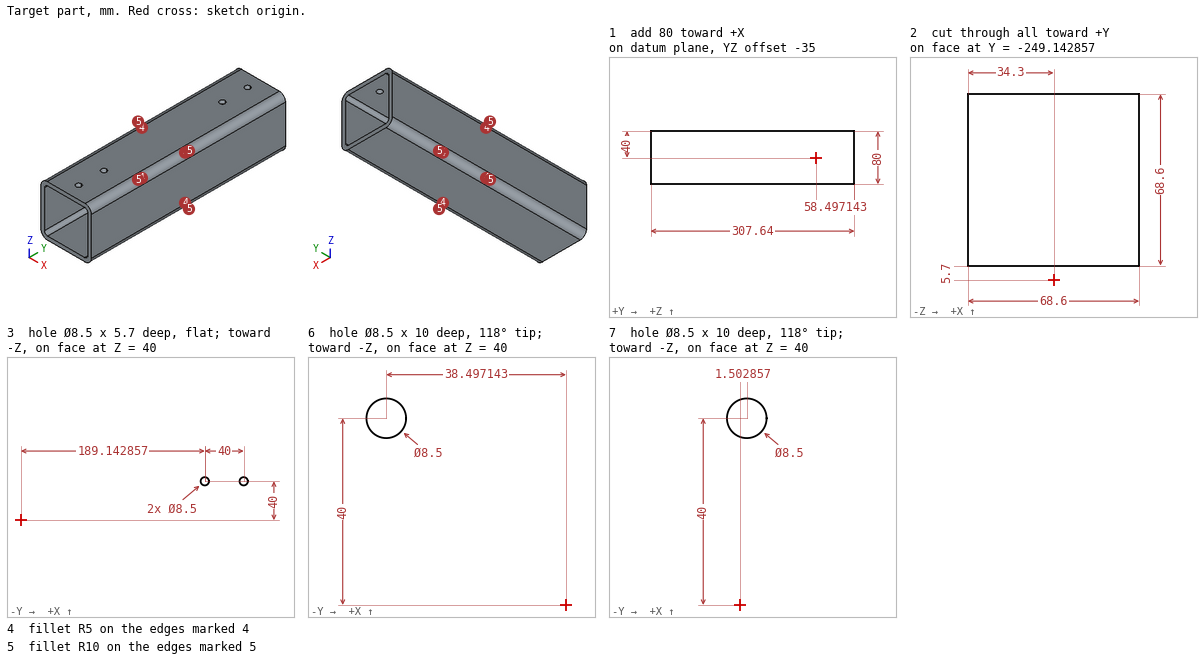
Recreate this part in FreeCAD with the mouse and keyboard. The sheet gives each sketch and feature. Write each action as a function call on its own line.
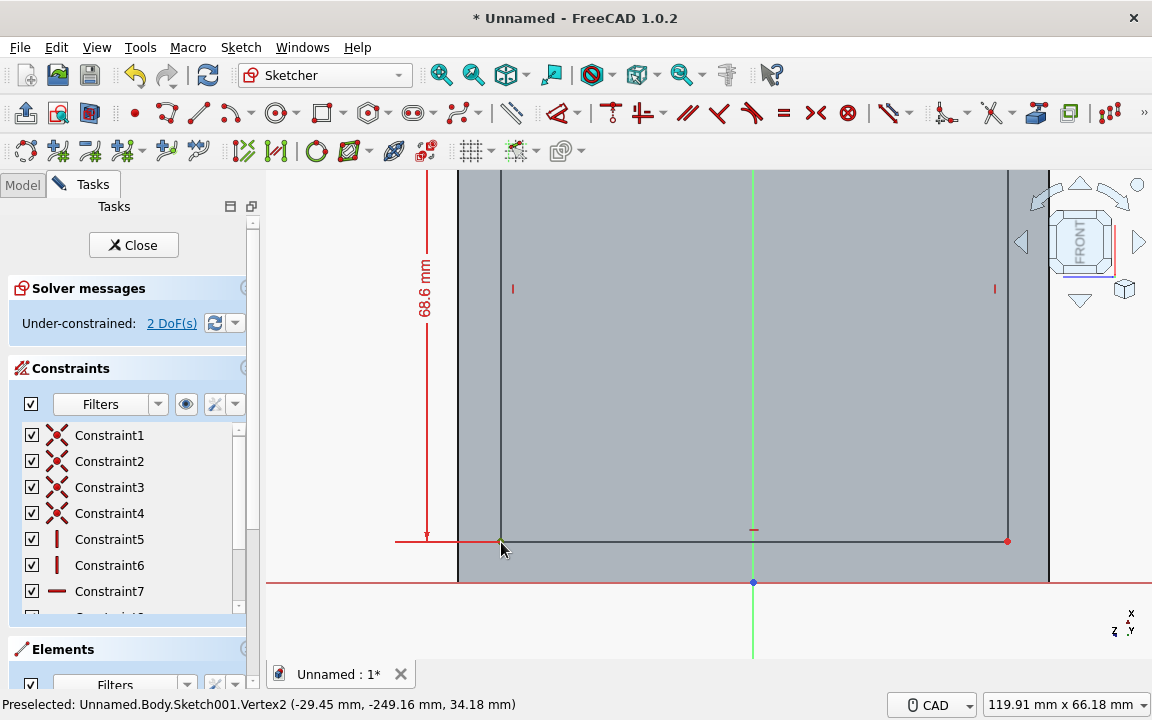
click(580, 114)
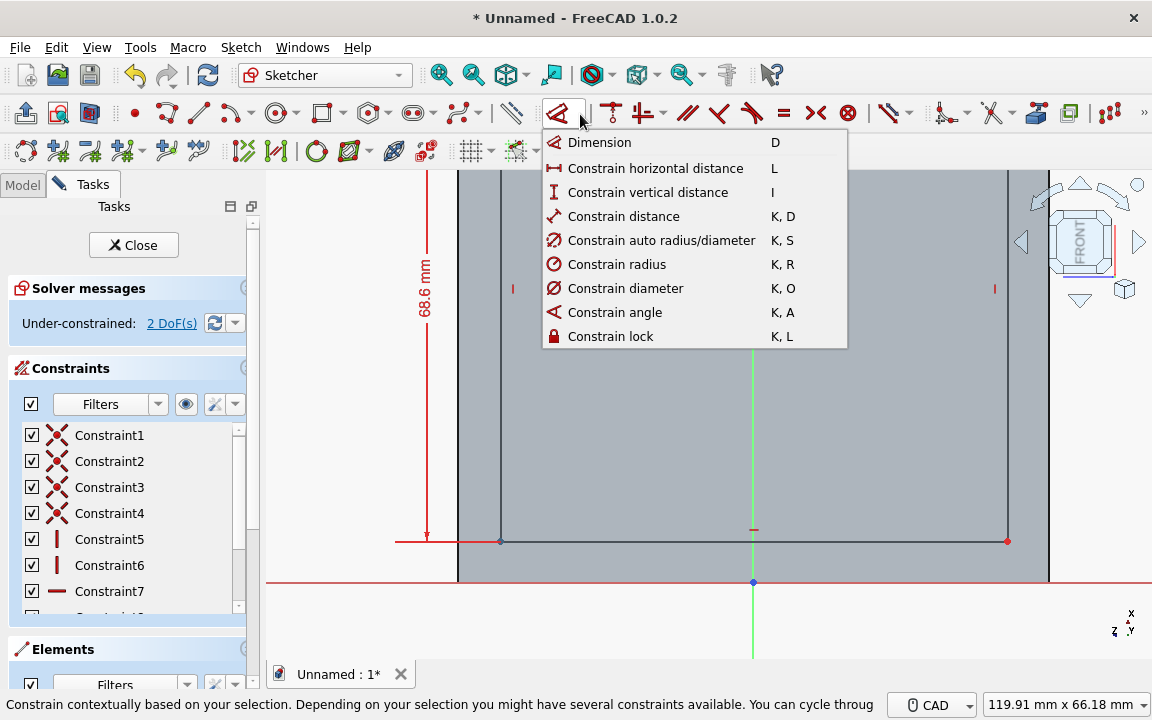
click(695, 192)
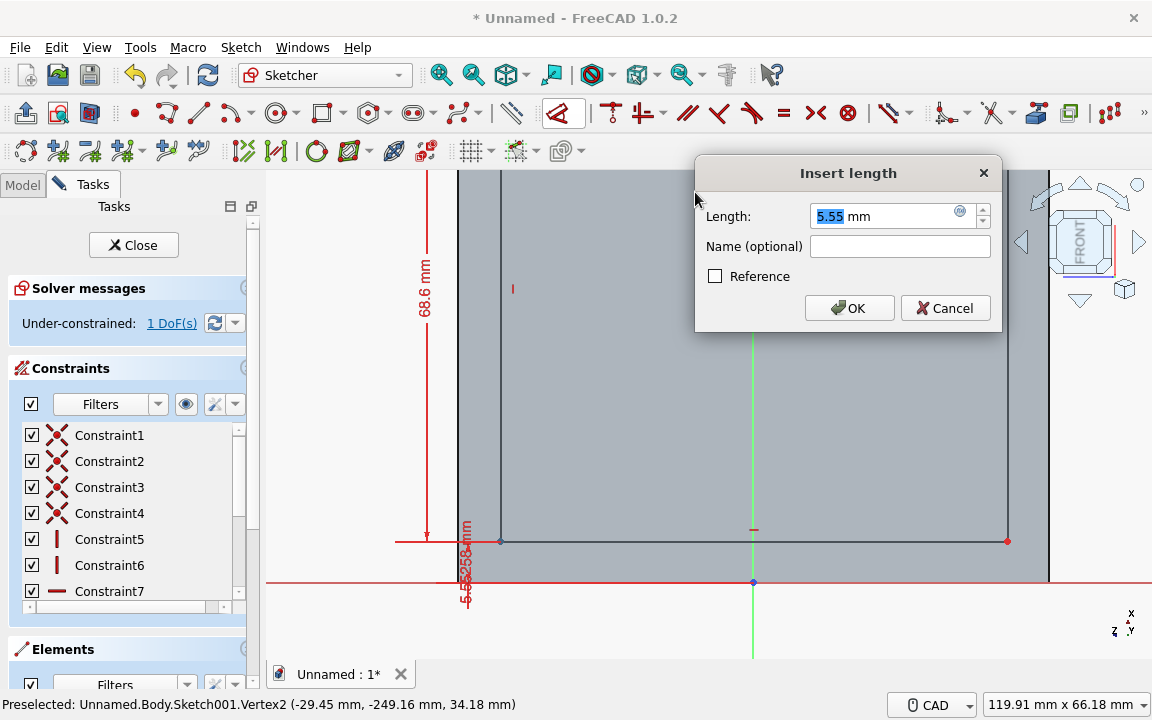
text(5.7)
key(Return)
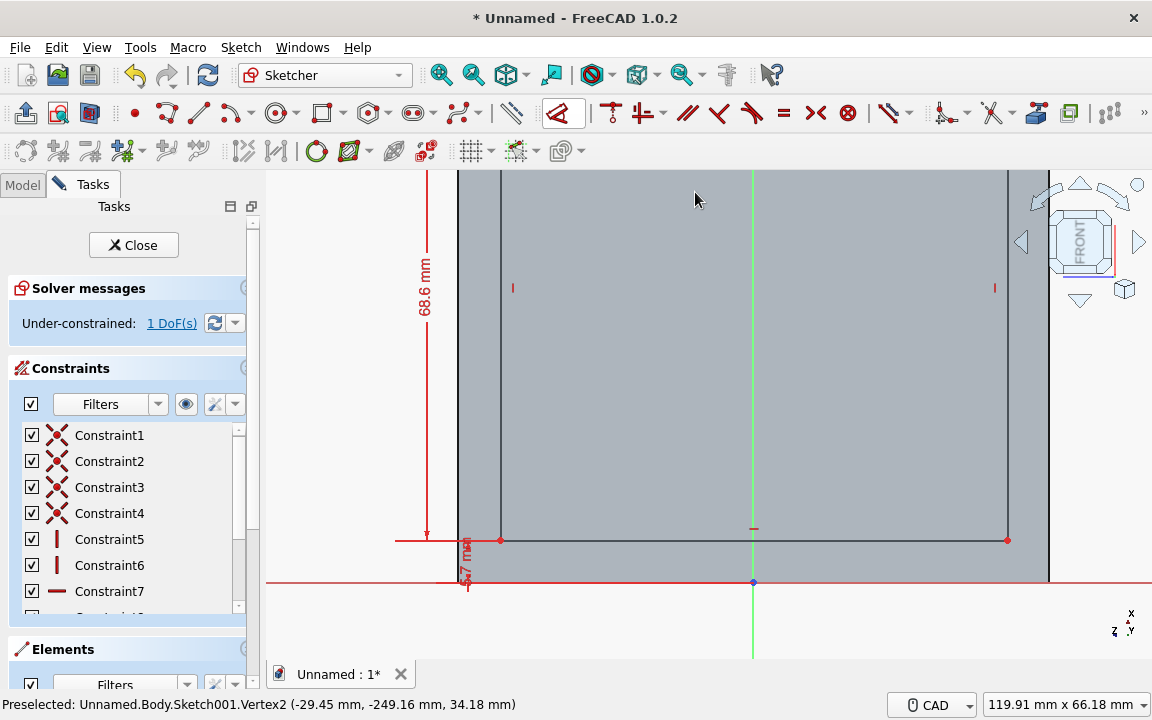
scroll(503, 544, down, 3)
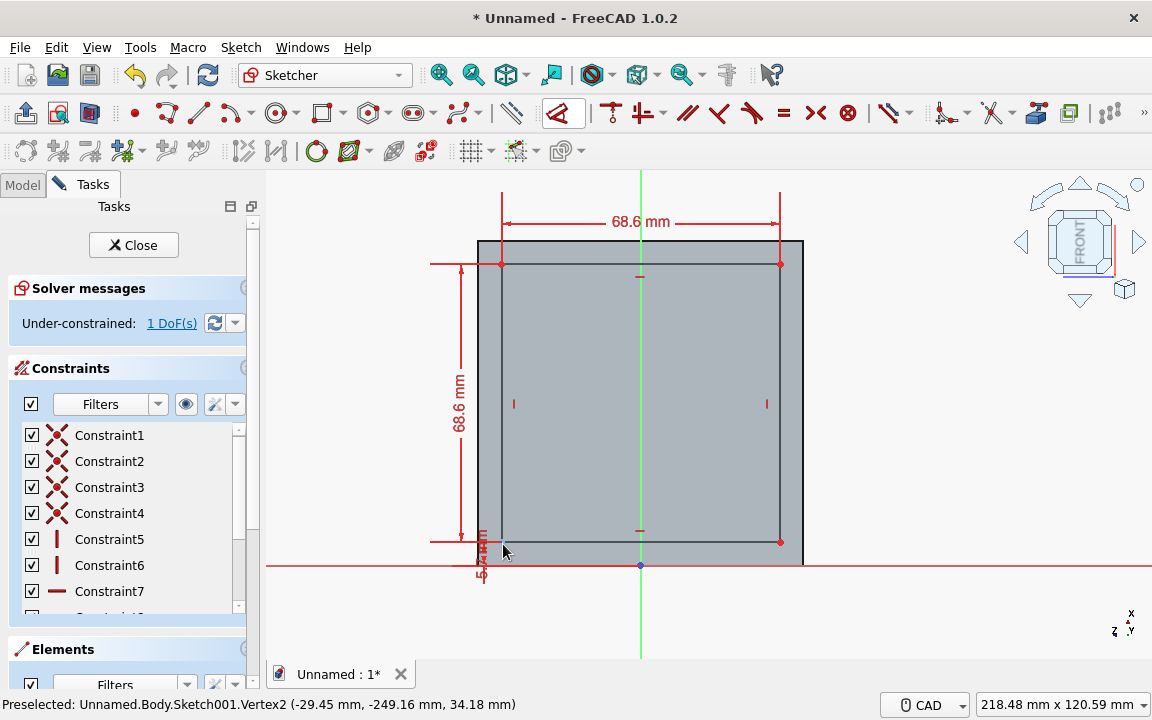
click(502, 264)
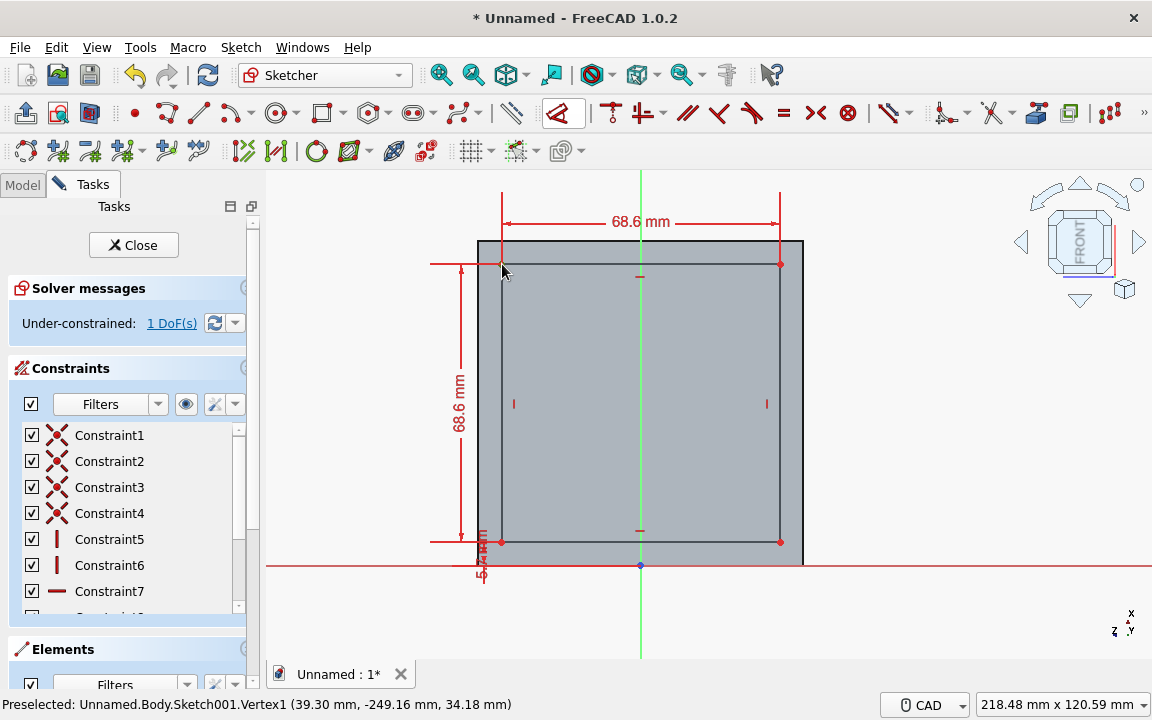
key(l)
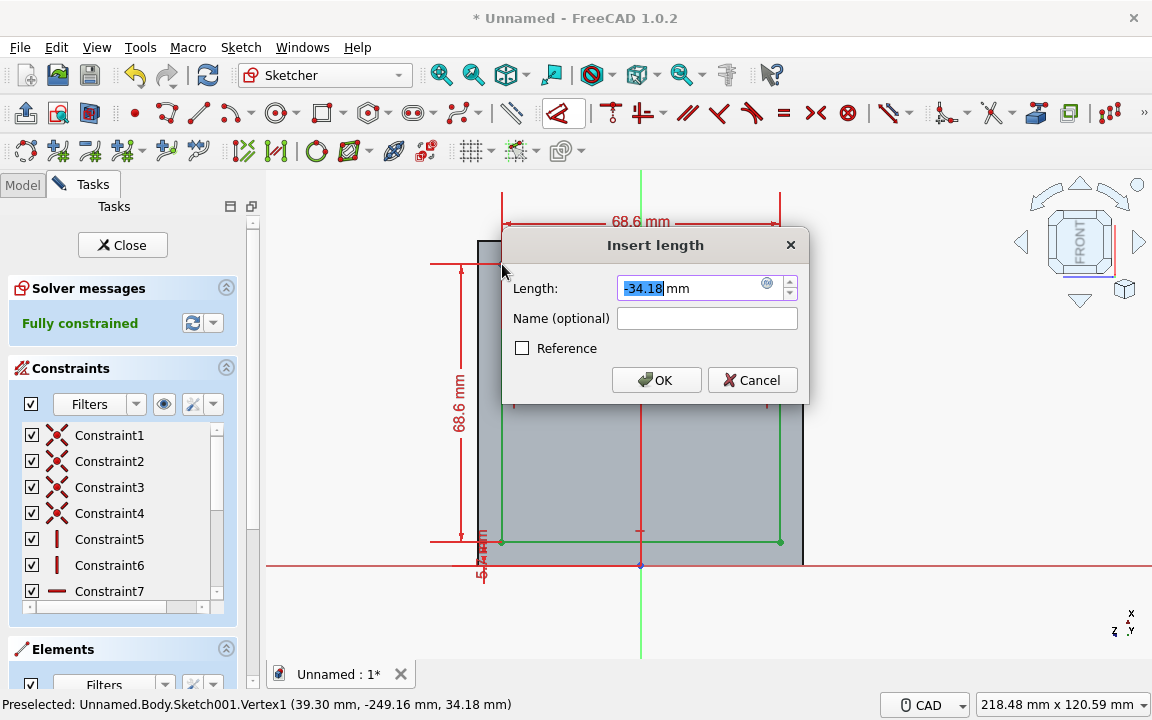
text(-34.3)
key(Return)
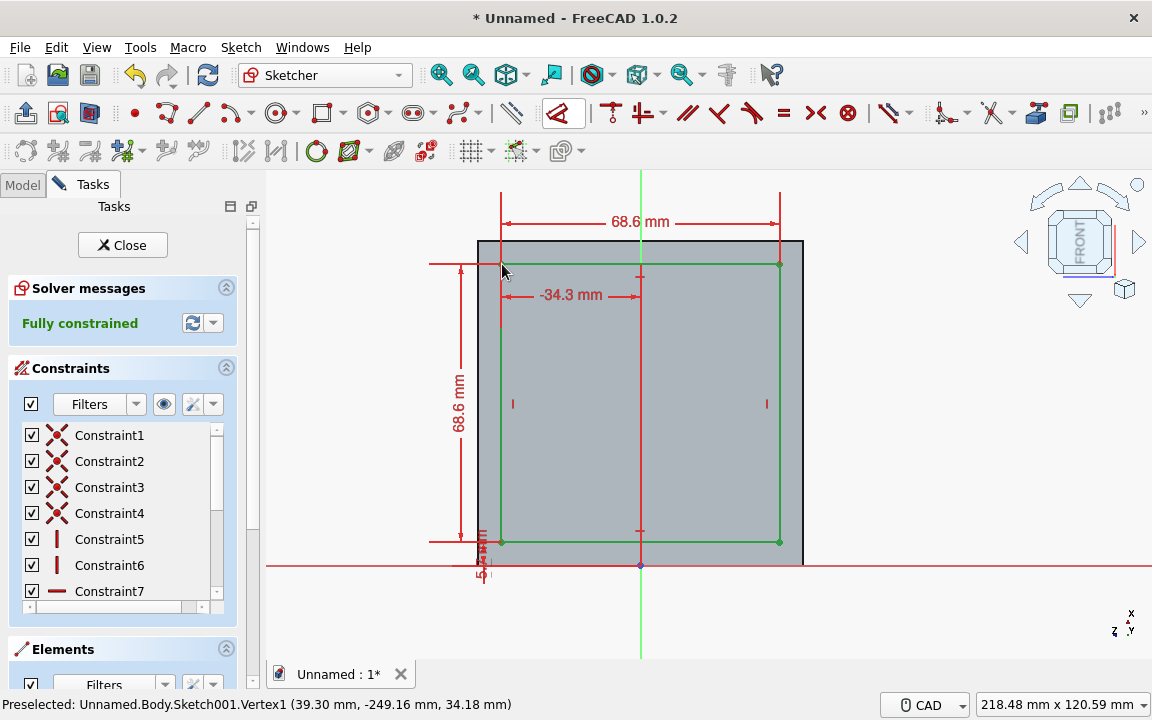
click(123, 245)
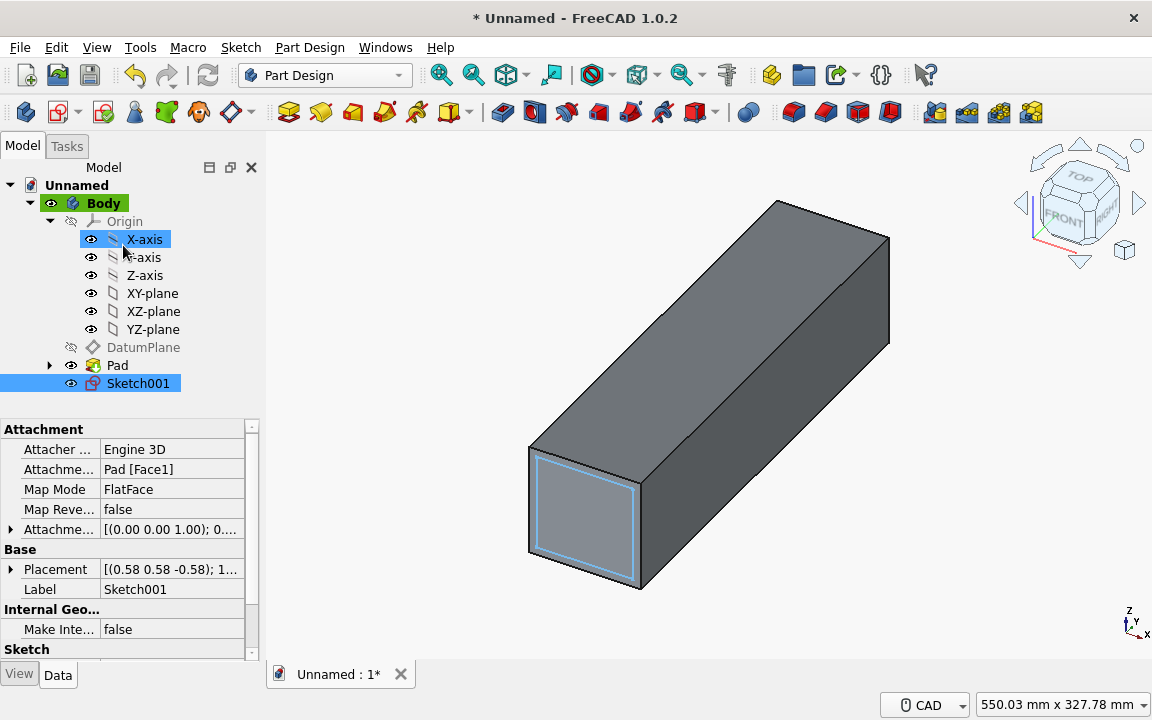
click(504, 112)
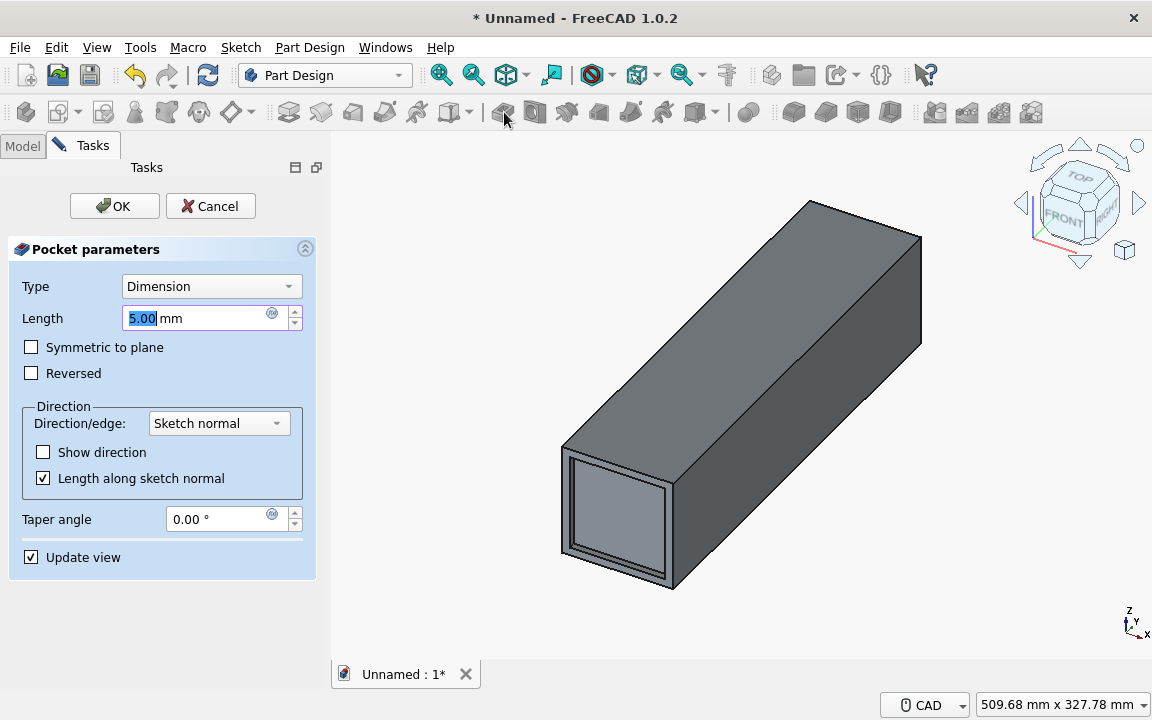
click(212, 286)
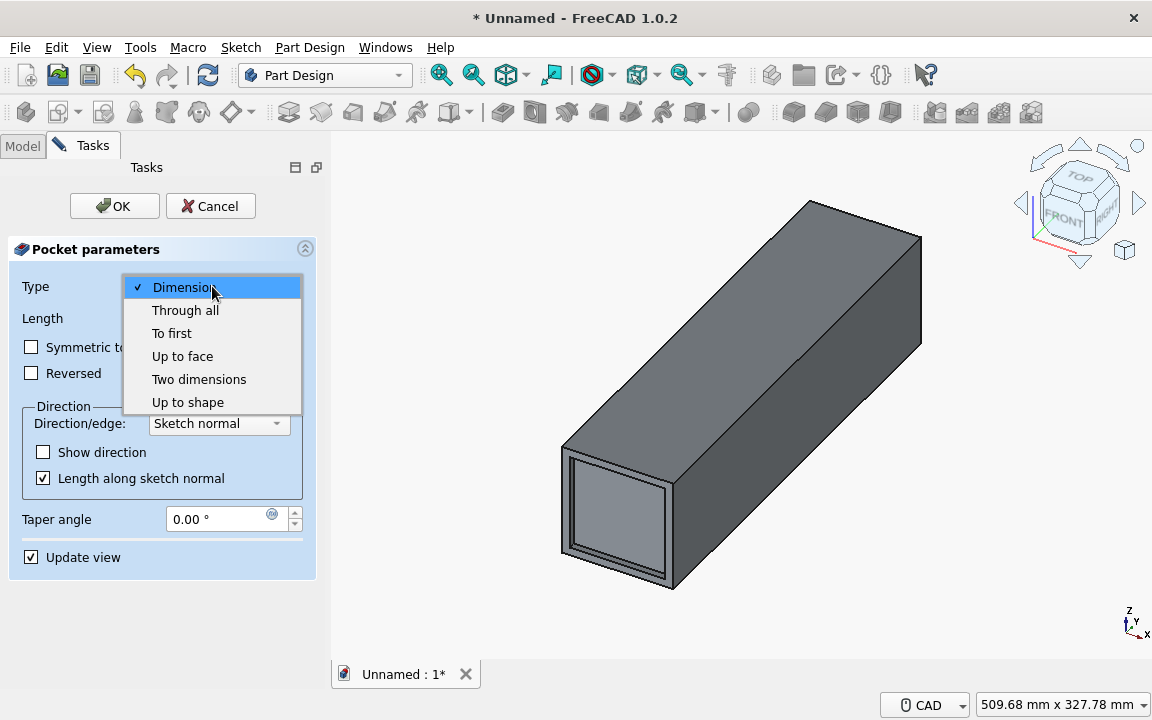
click(212, 310)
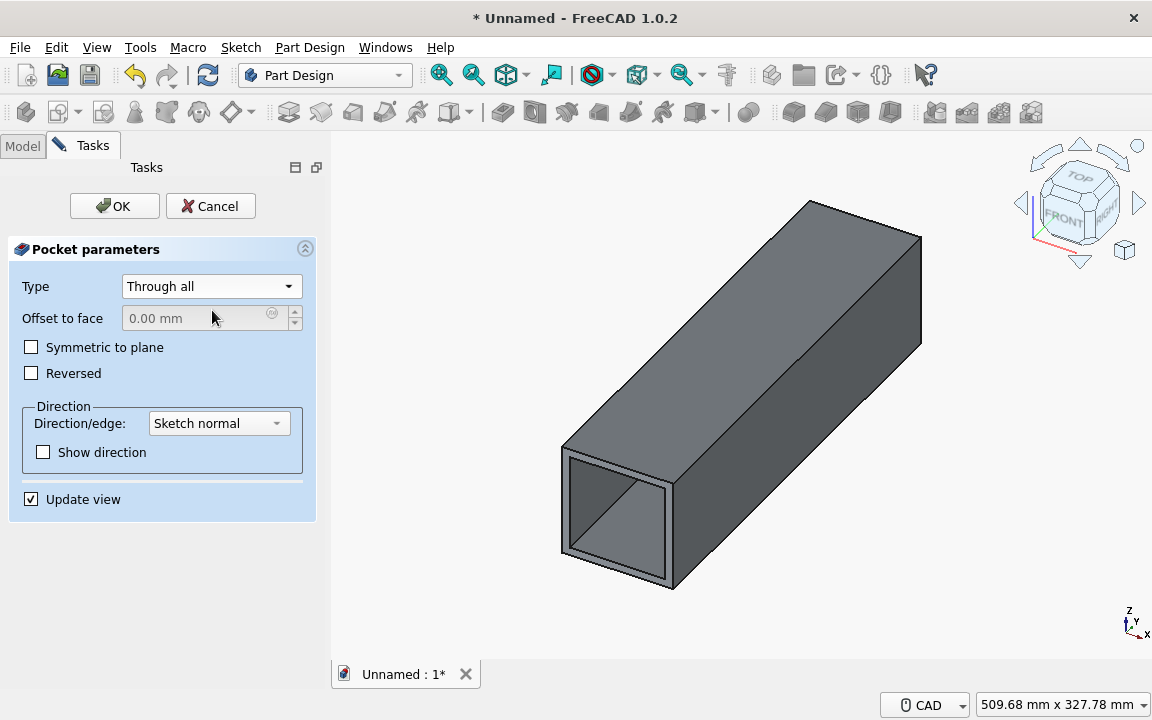
click(115, 206)